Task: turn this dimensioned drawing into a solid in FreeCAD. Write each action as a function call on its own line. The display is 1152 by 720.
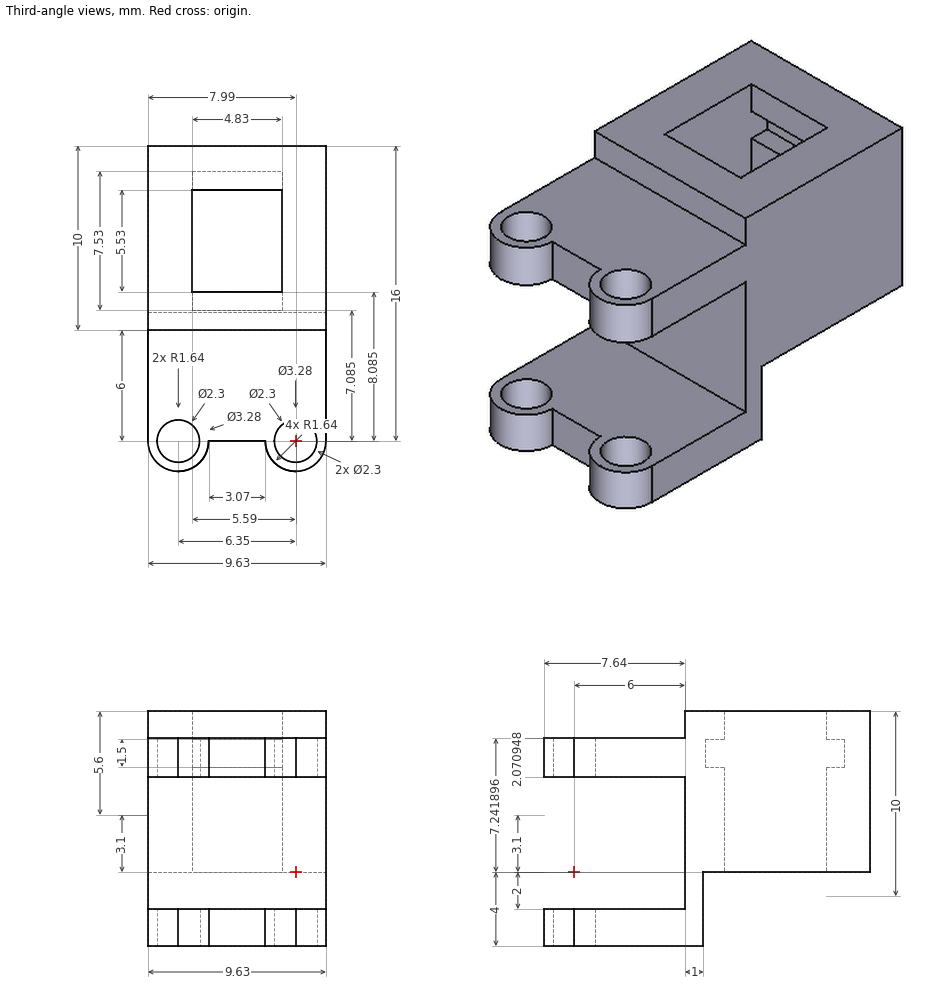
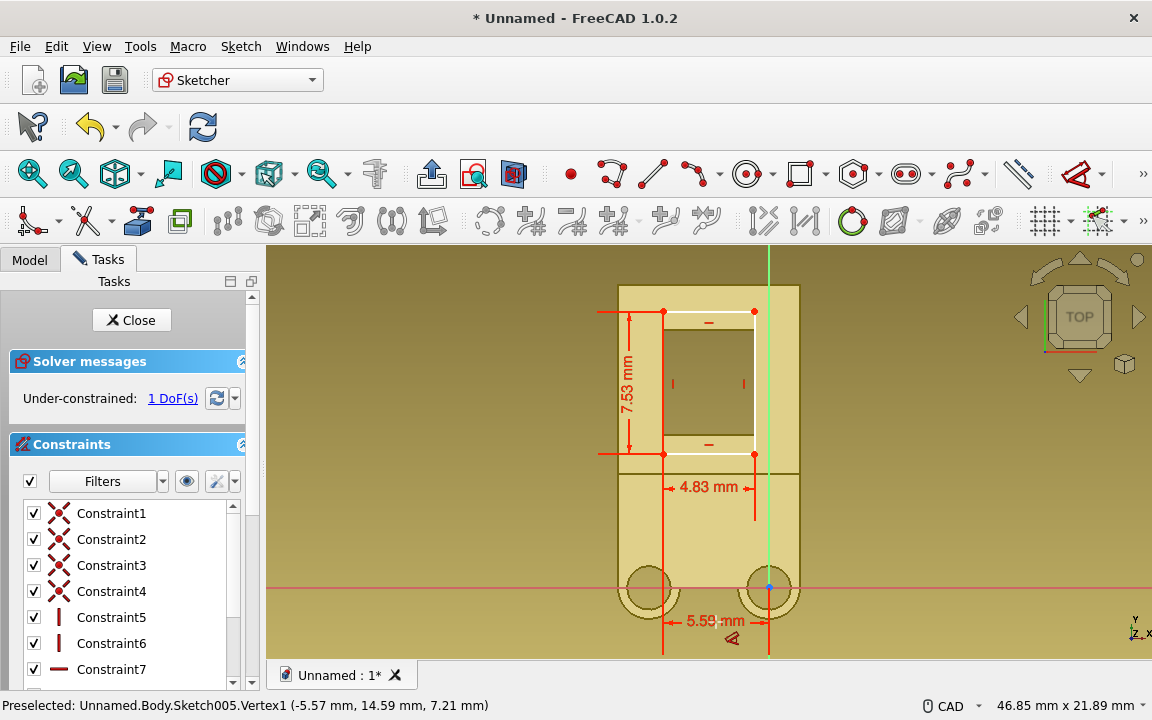
click(663, 454)
click(803, 521)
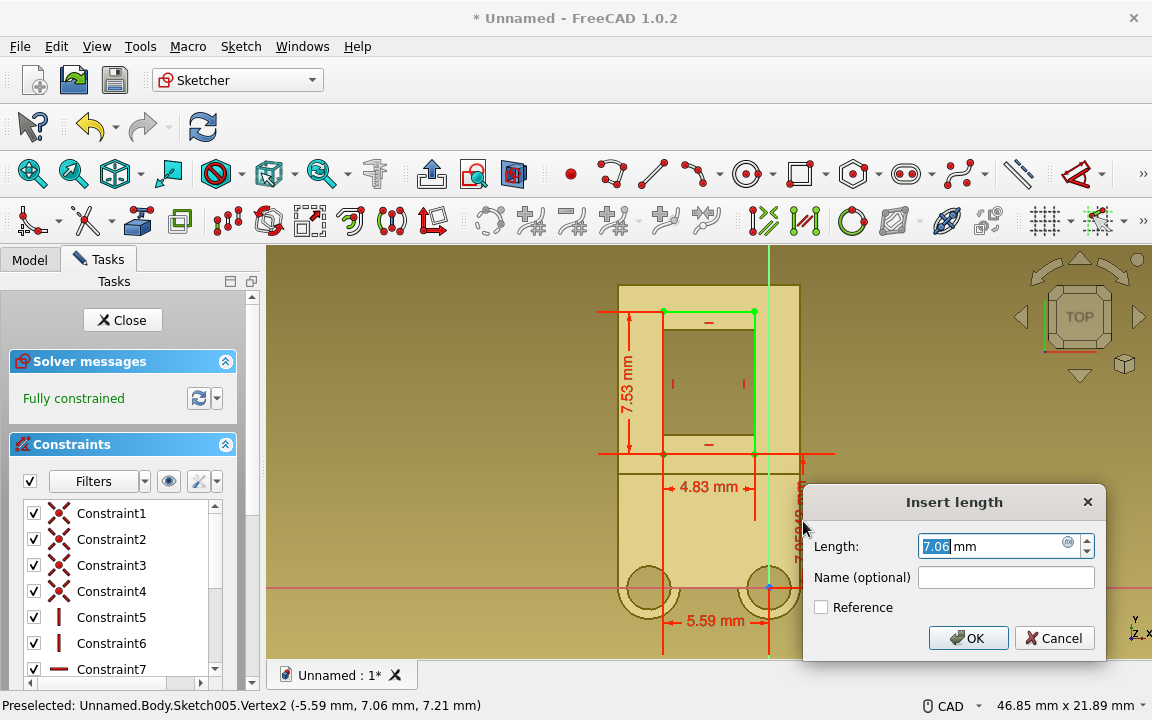
text(7.085)
key(Return)
key(Escape)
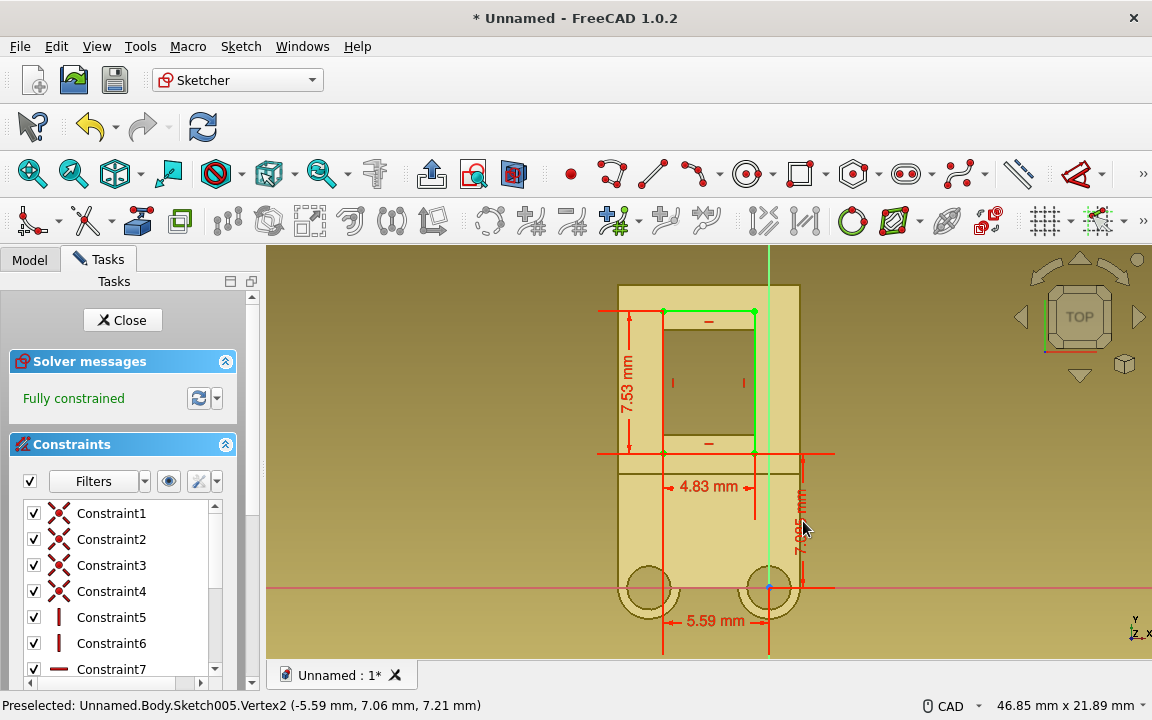
click(123, 320)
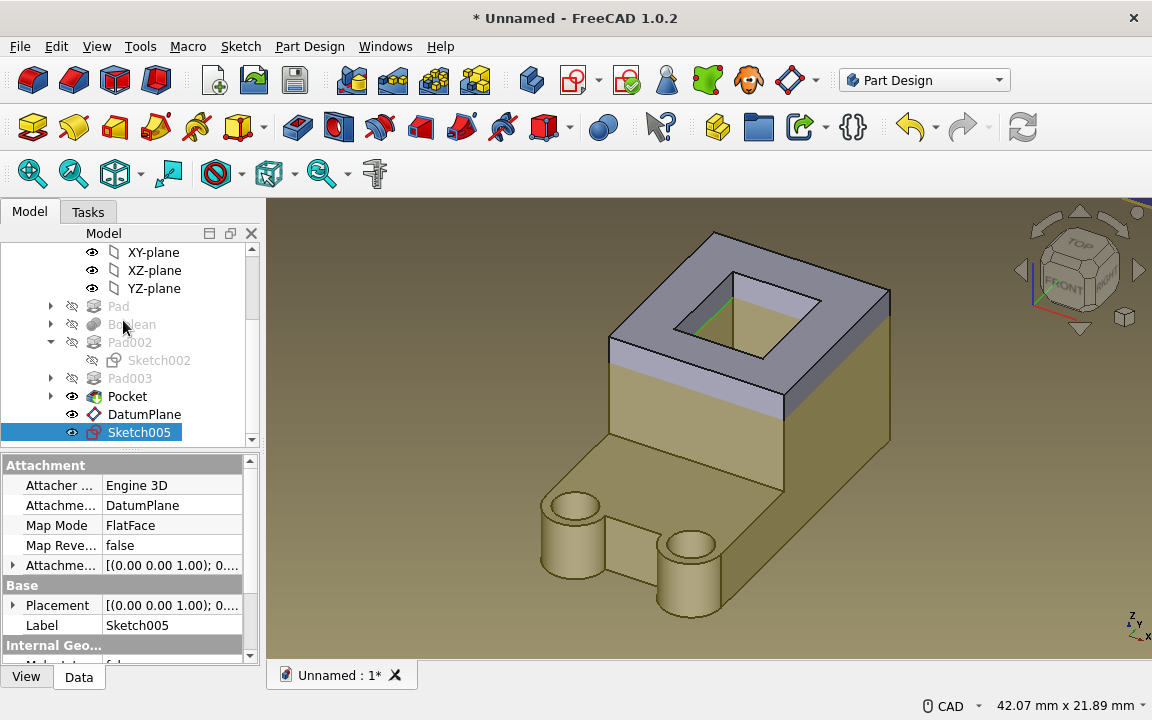
click(298, 128)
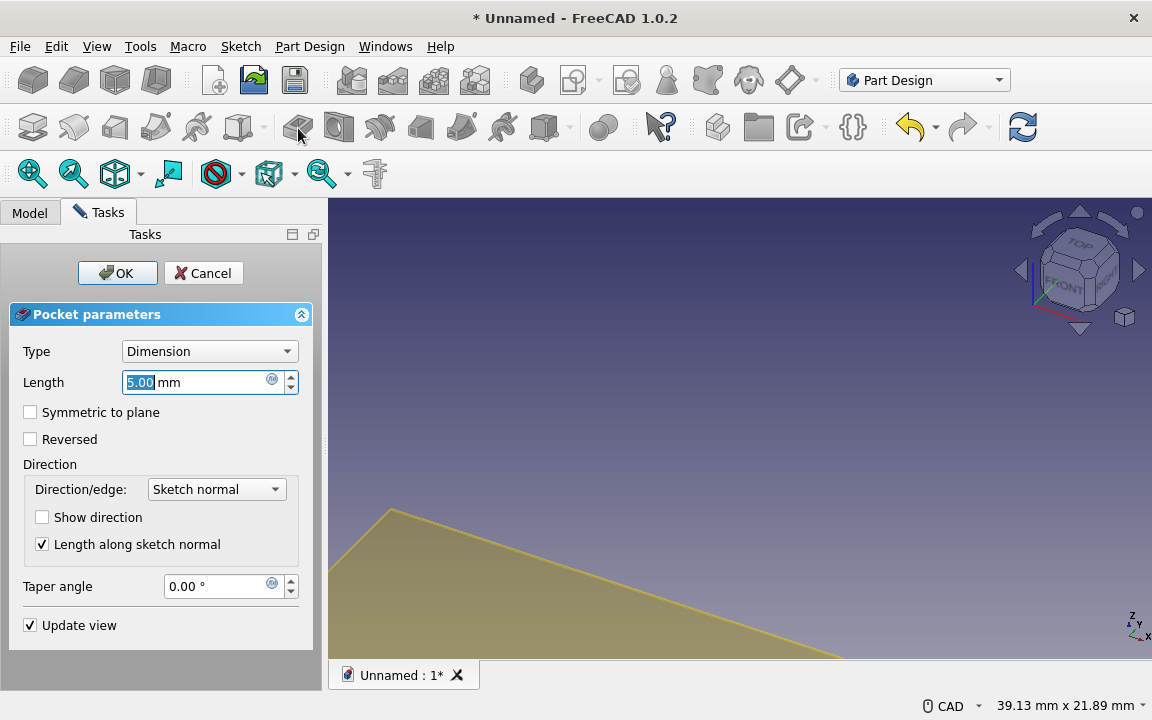
text(1.5)
key(Tab)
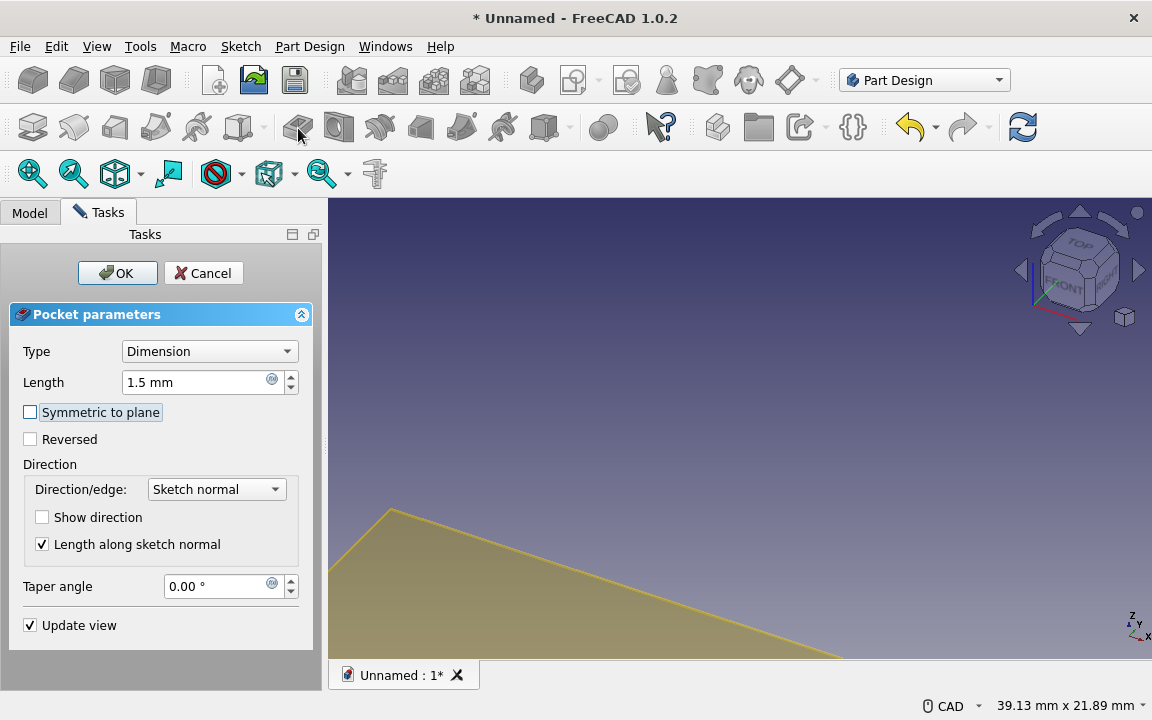
click(118, 273)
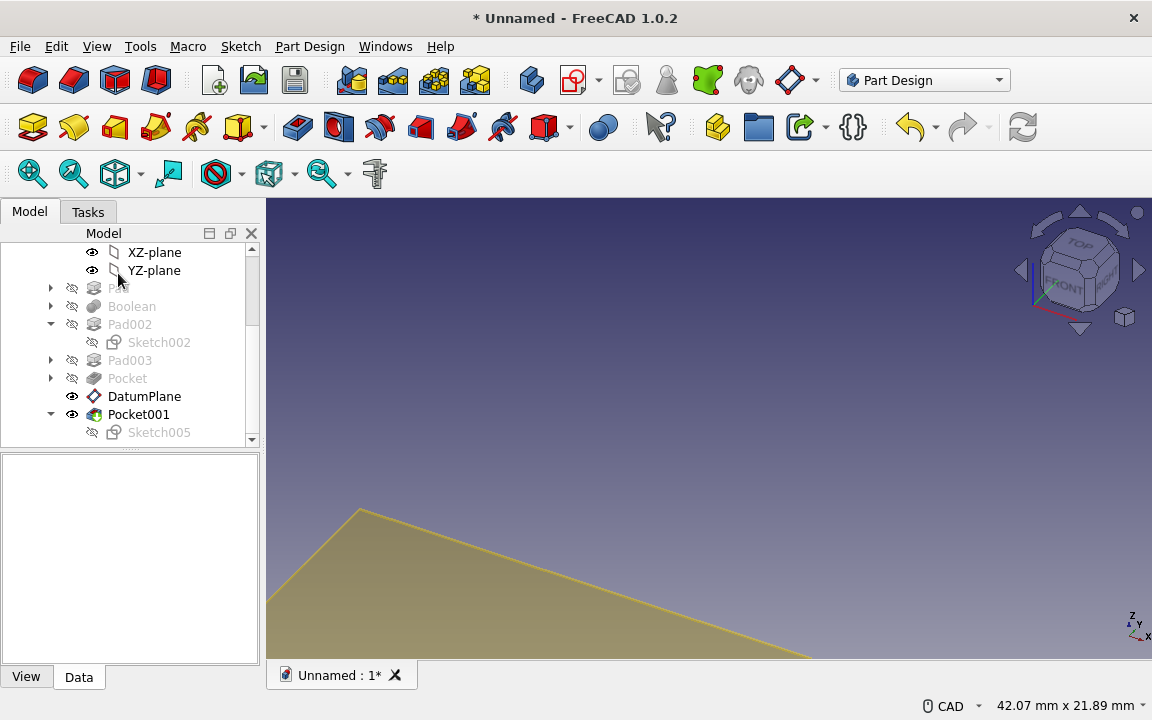
click(117, 396)
key(space)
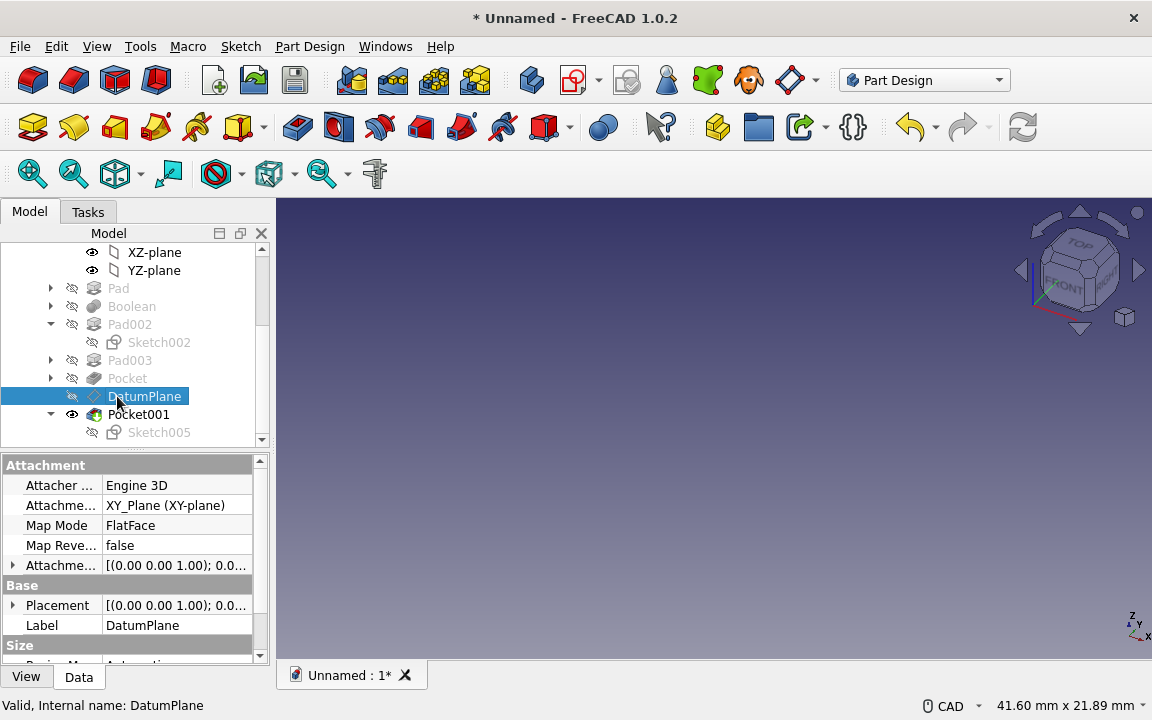
click(33, 174)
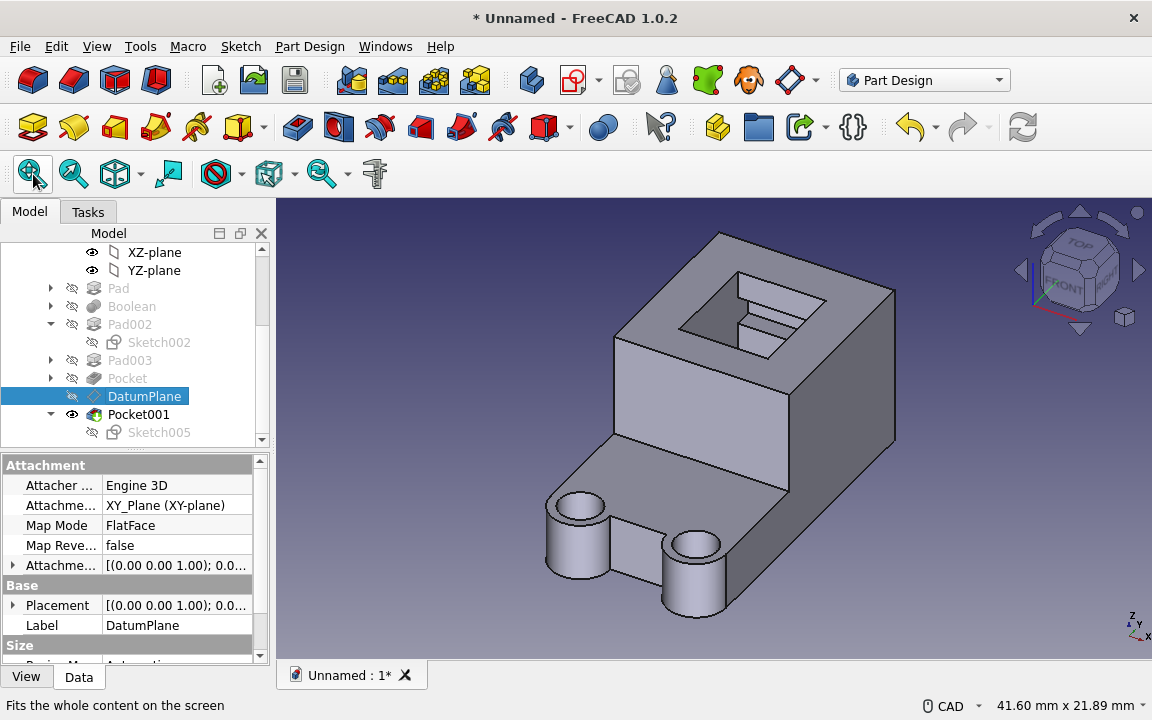
key(6)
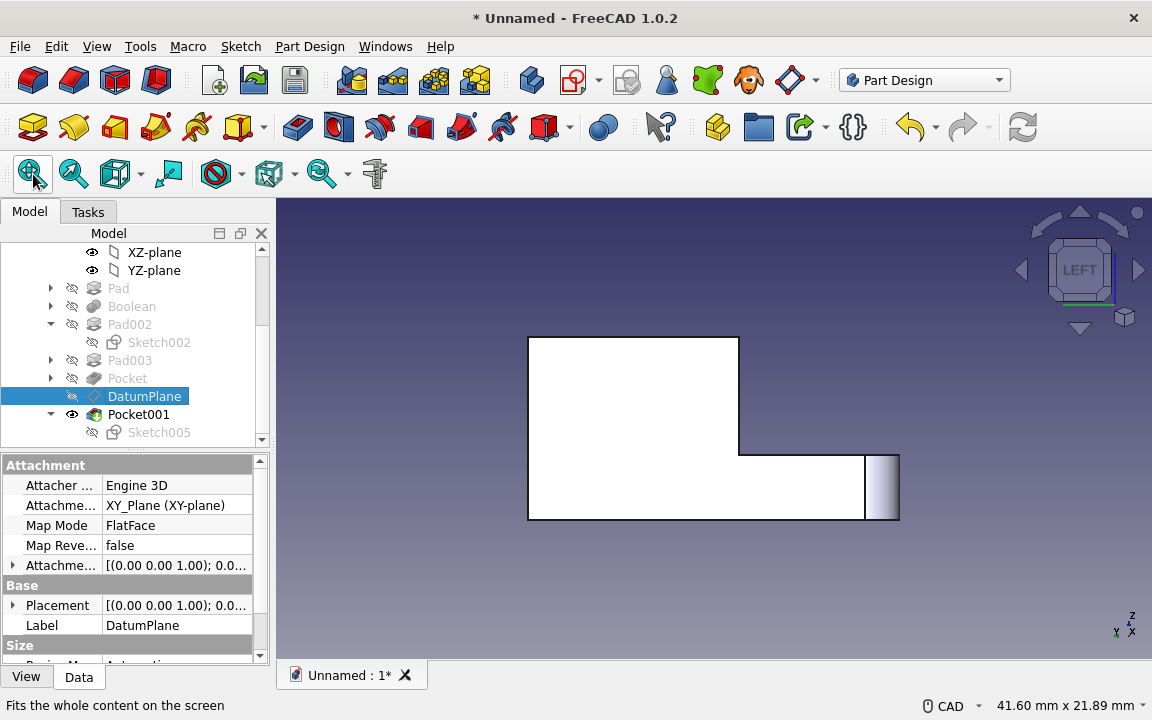
click(33, 174)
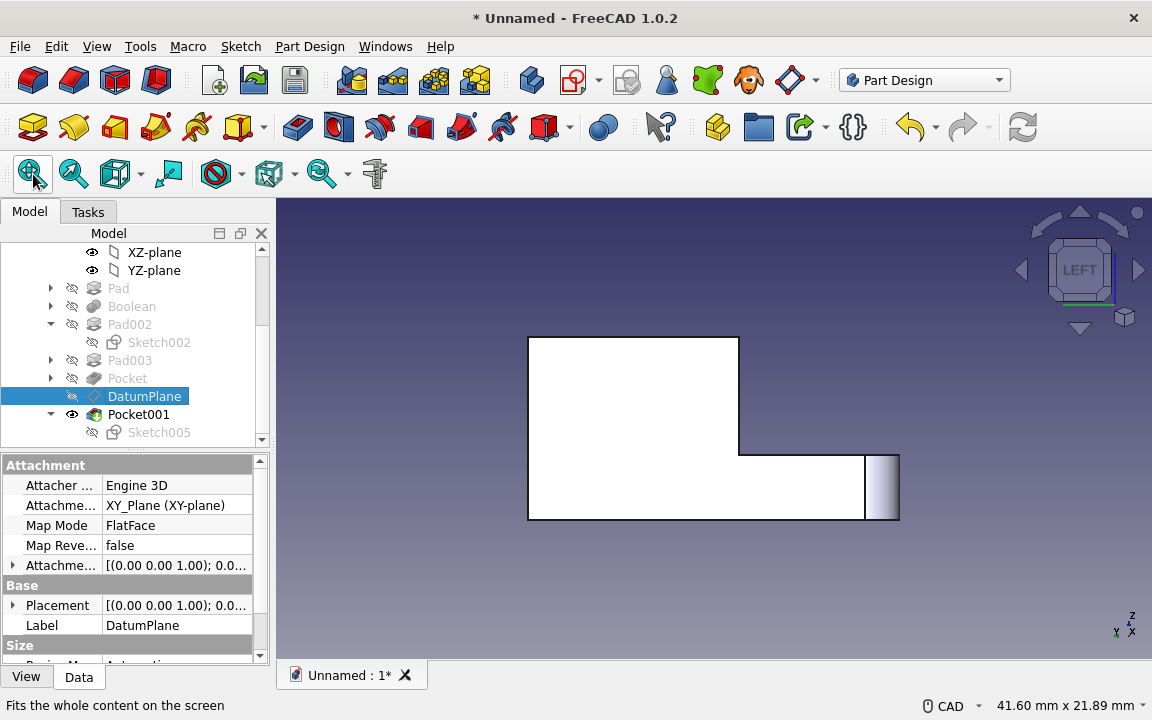
click(649, 427)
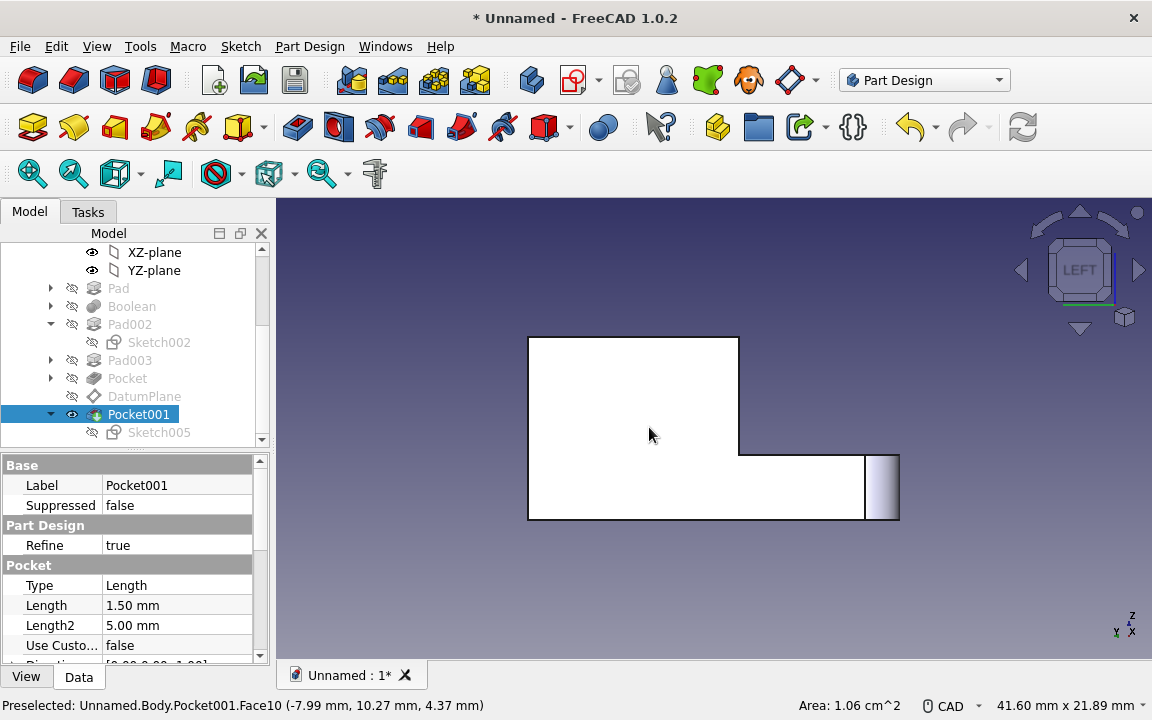
click(572, 80)